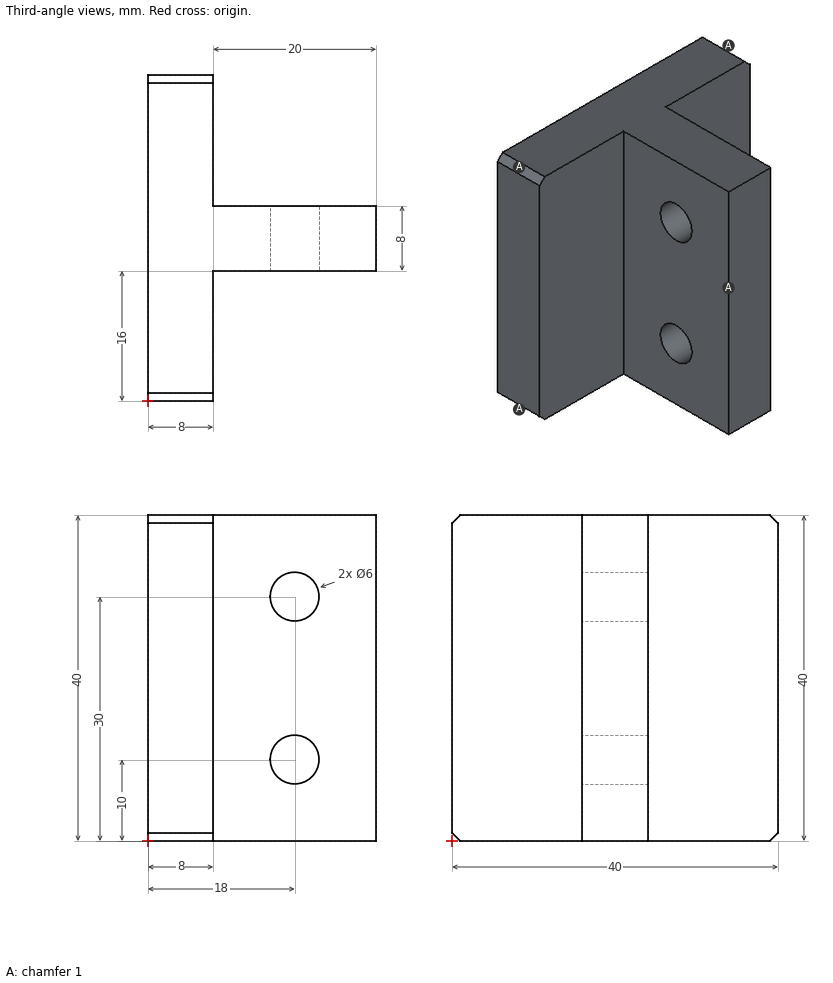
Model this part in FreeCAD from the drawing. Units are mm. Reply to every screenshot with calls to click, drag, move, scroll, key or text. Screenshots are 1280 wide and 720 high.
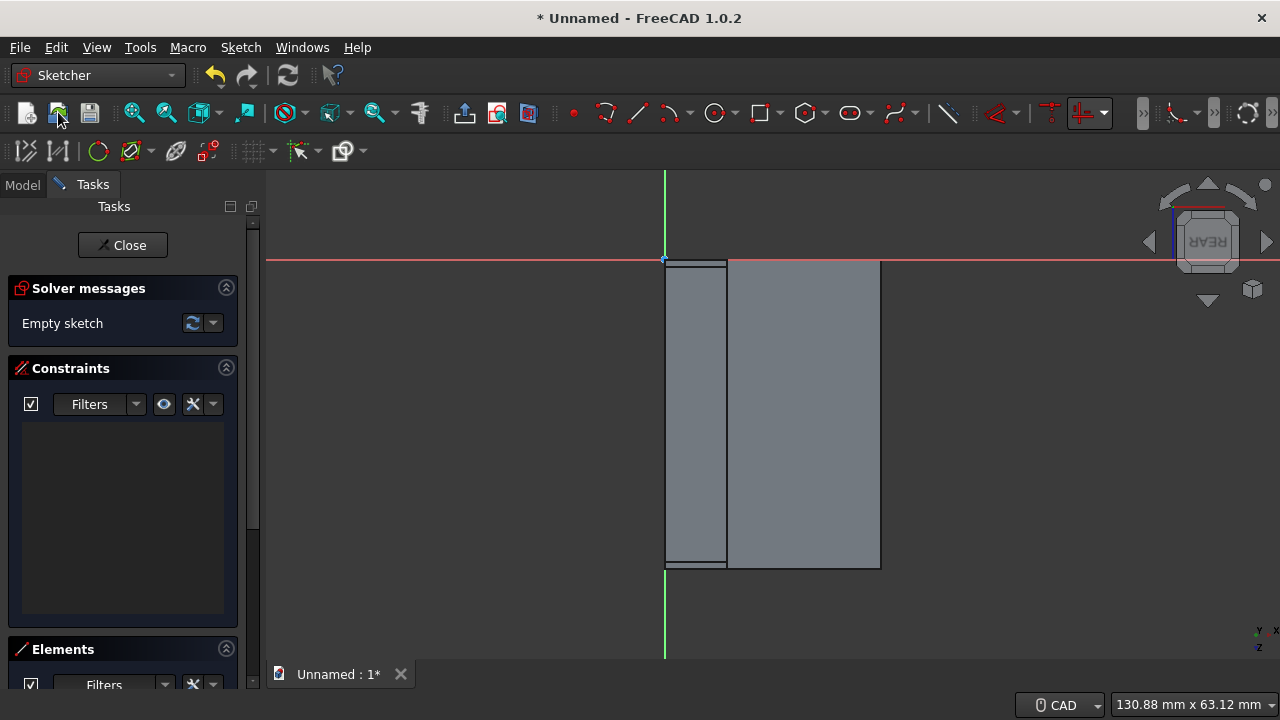
key(q)
key(s)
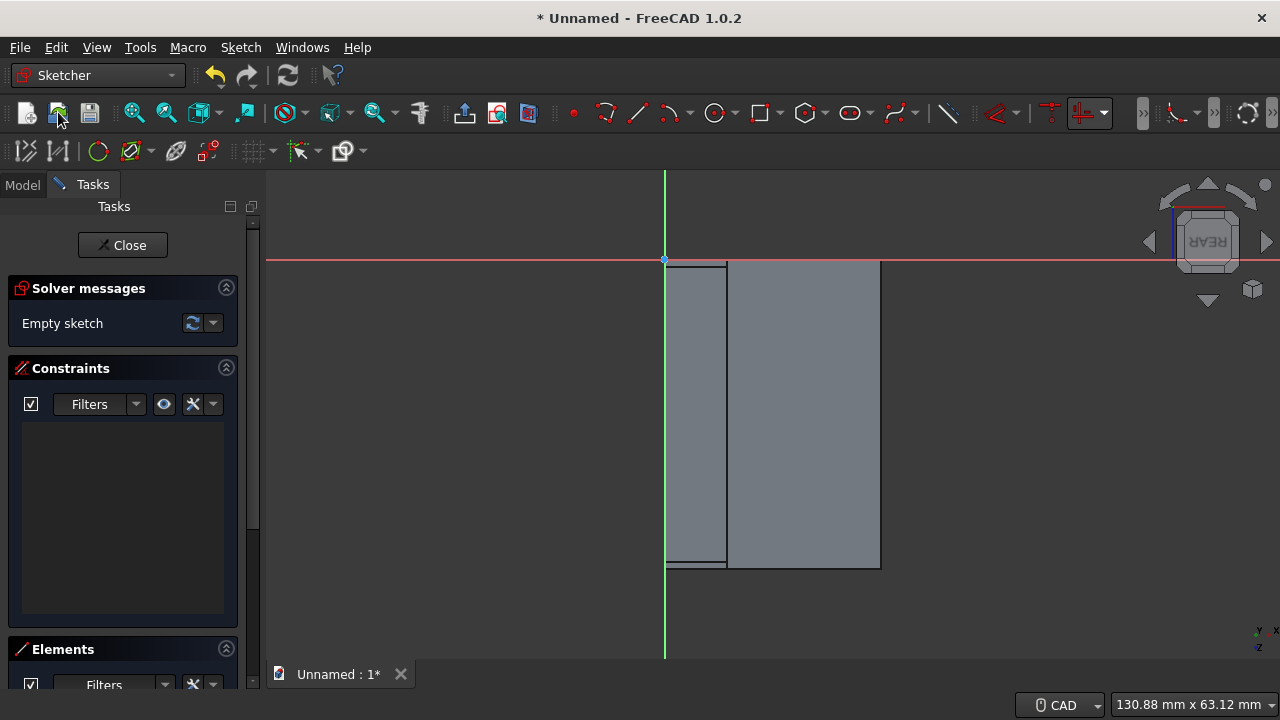
key(g)
key(c)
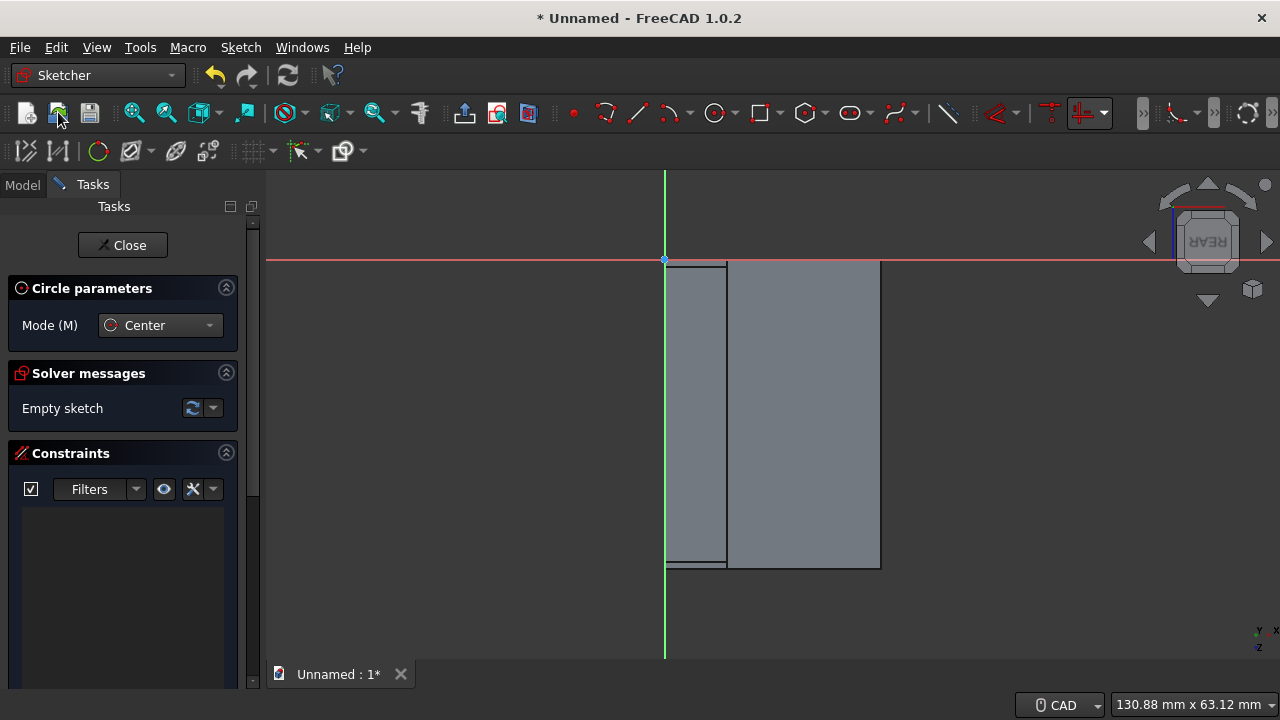
click(804, 492)
click(820, 476)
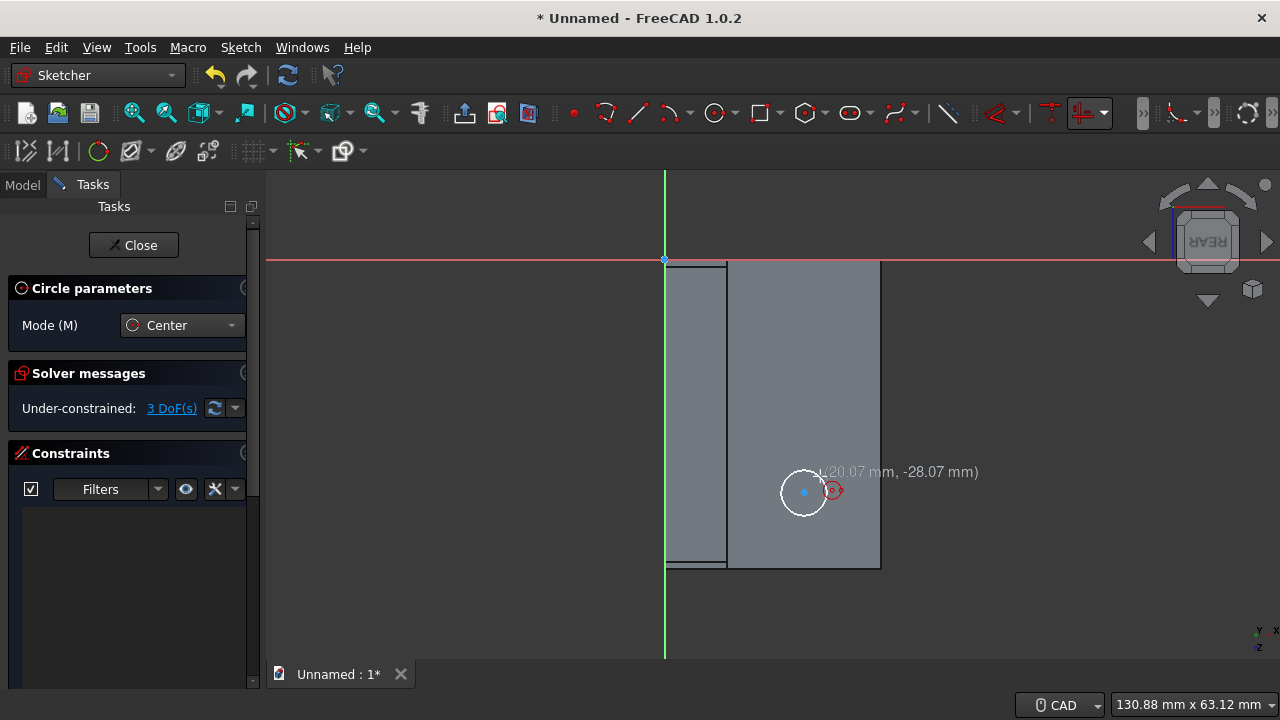
click(804, 337)
click(820, 321)
key(Escape)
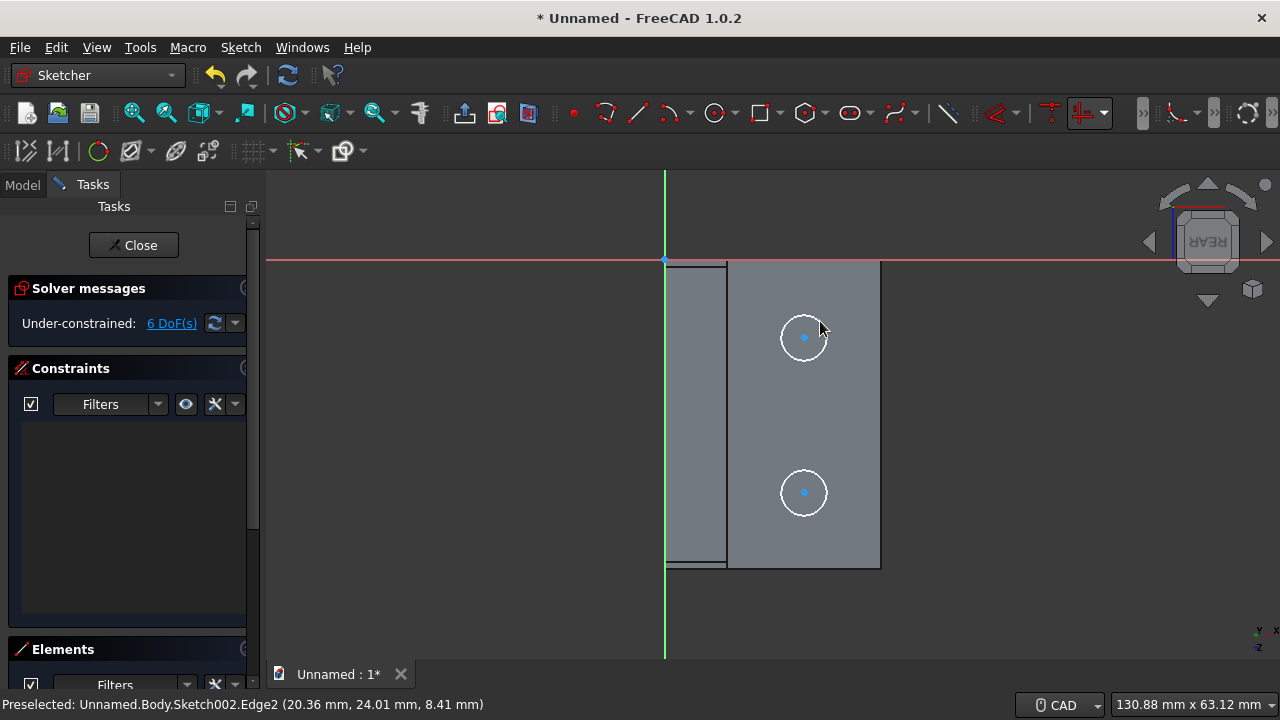
click(820, 477)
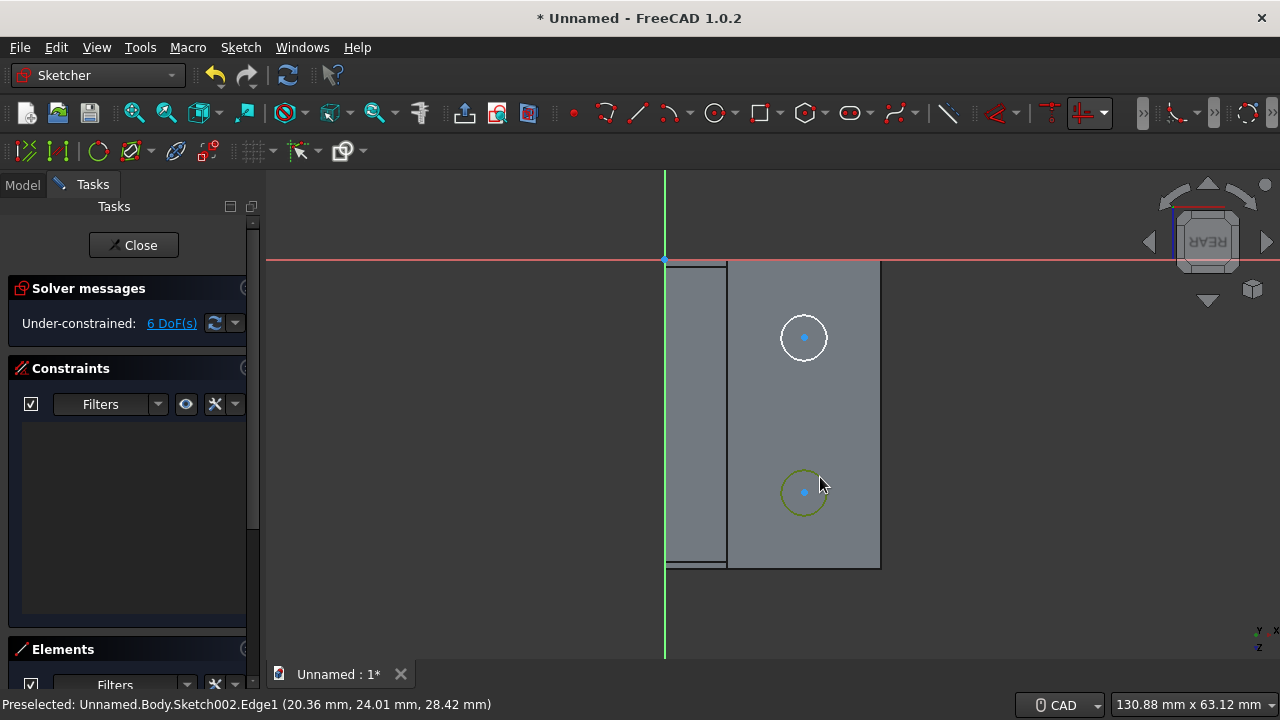
click(820, 322)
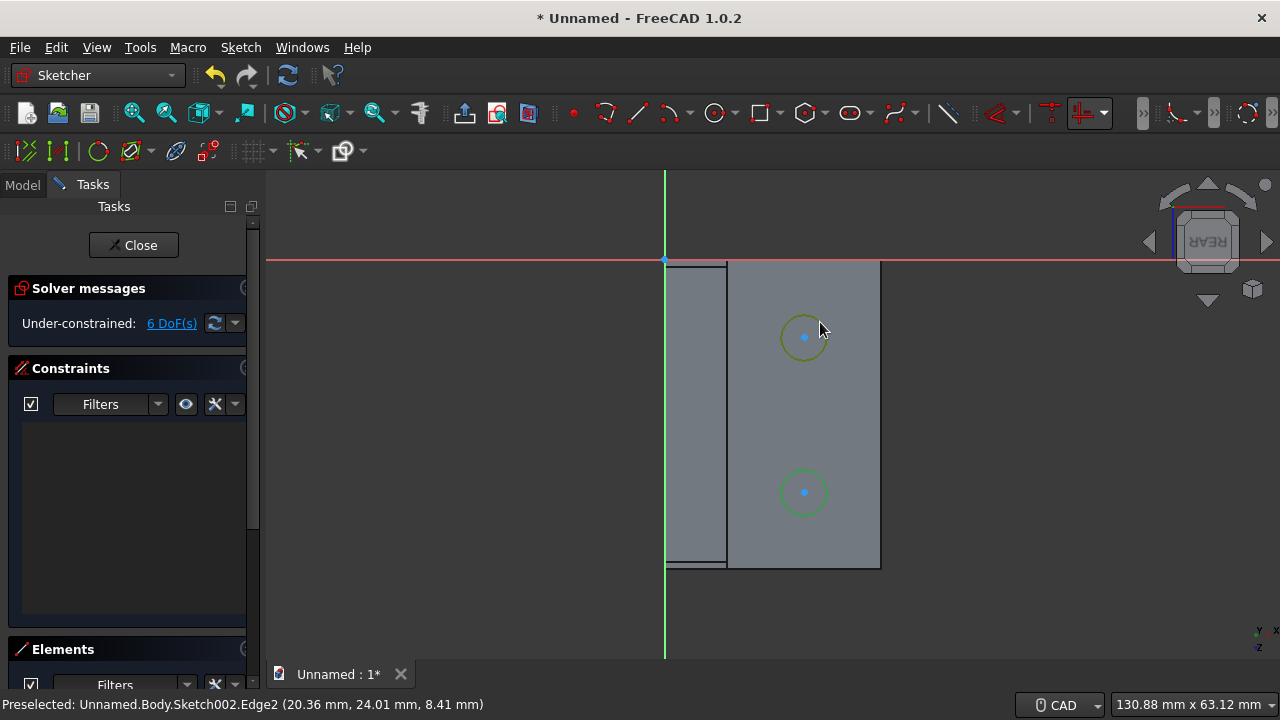
key(e)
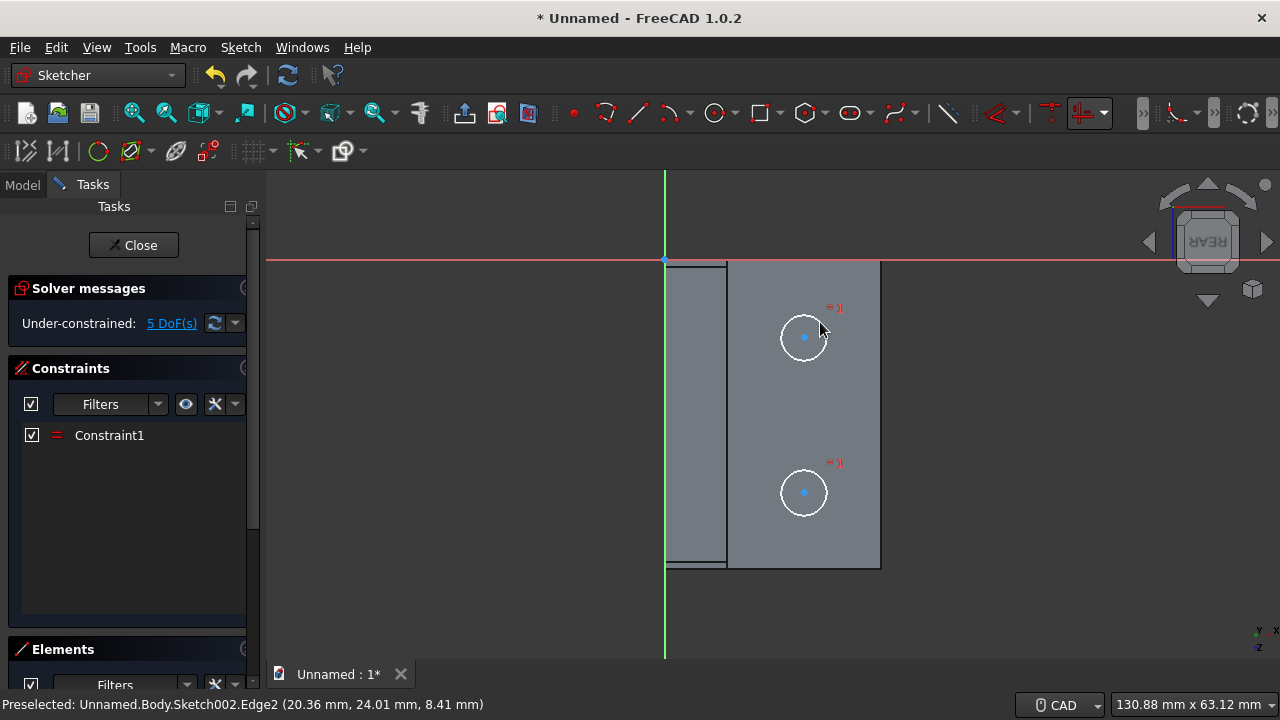
click(996, 114)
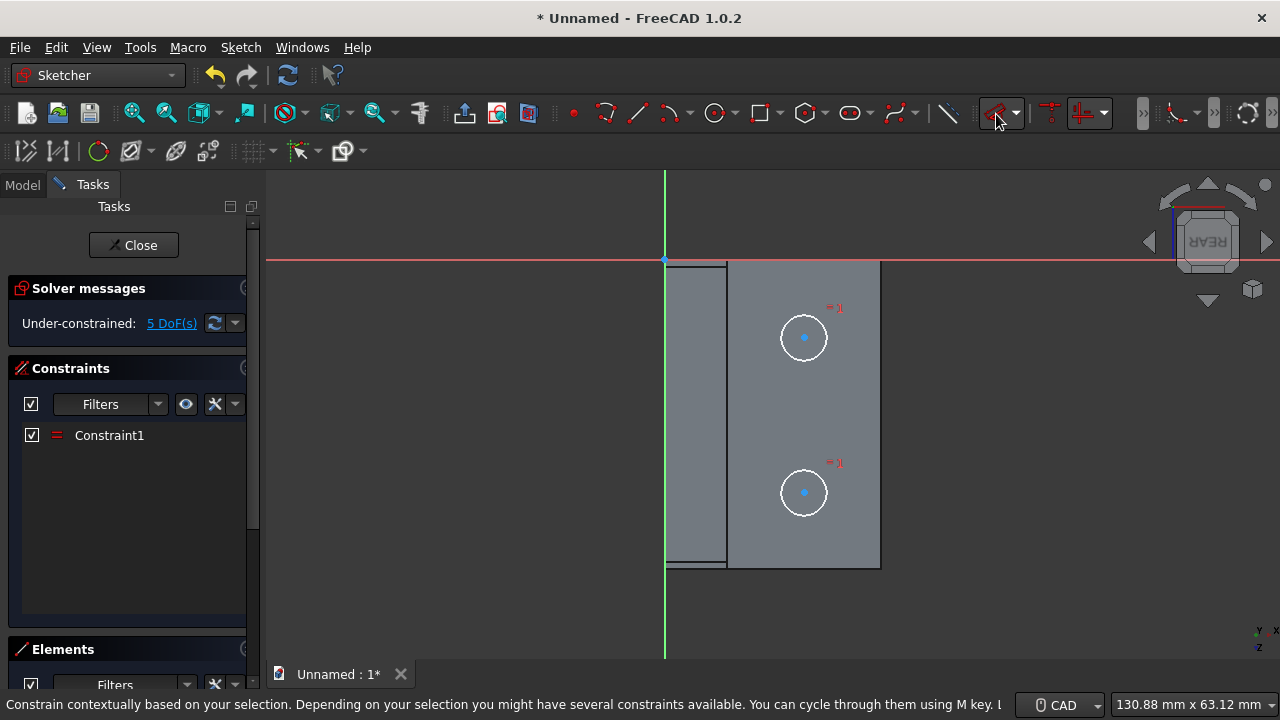
click(820, 477)
click(843, 454)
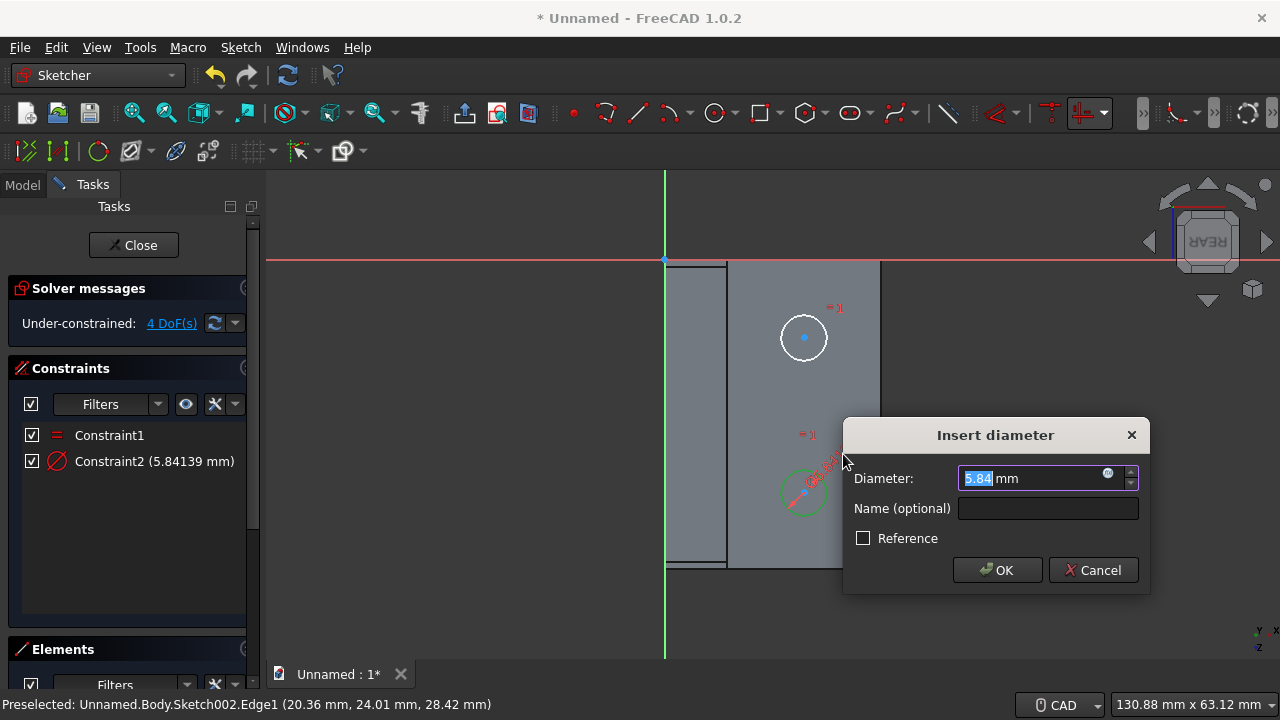
text(6)
key(Return)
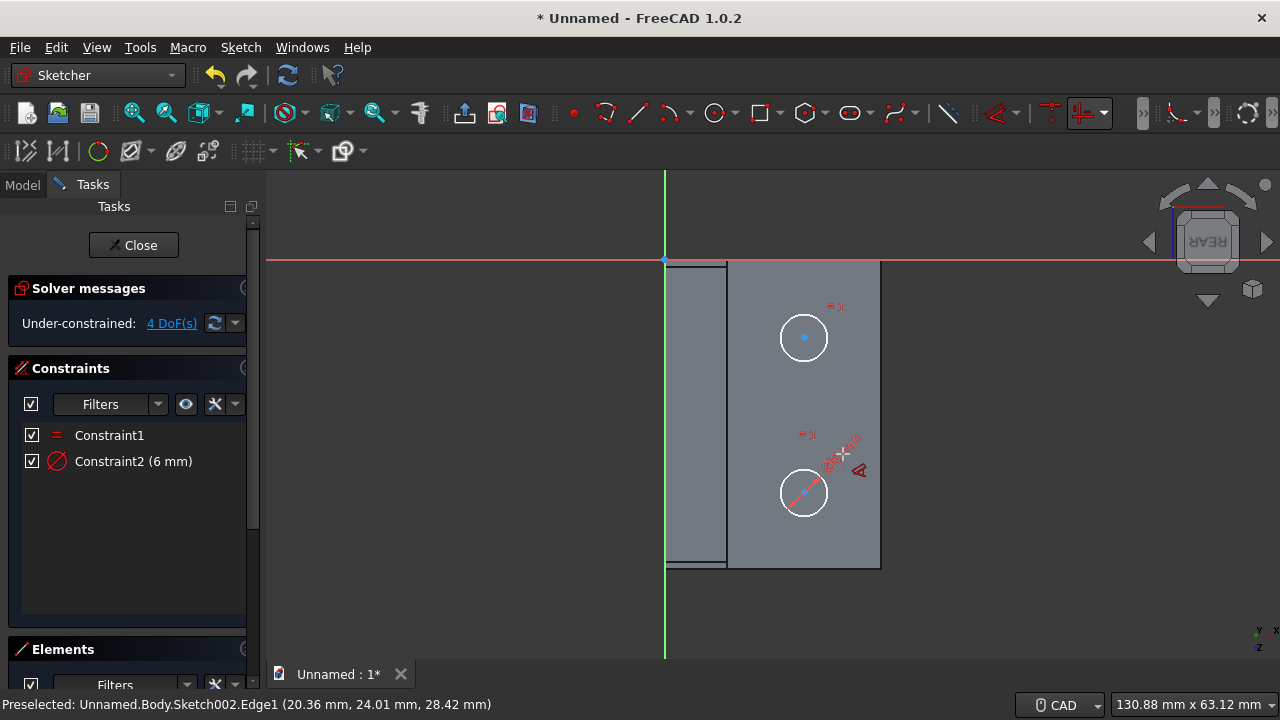
click(804, 493)
click(734, 226)